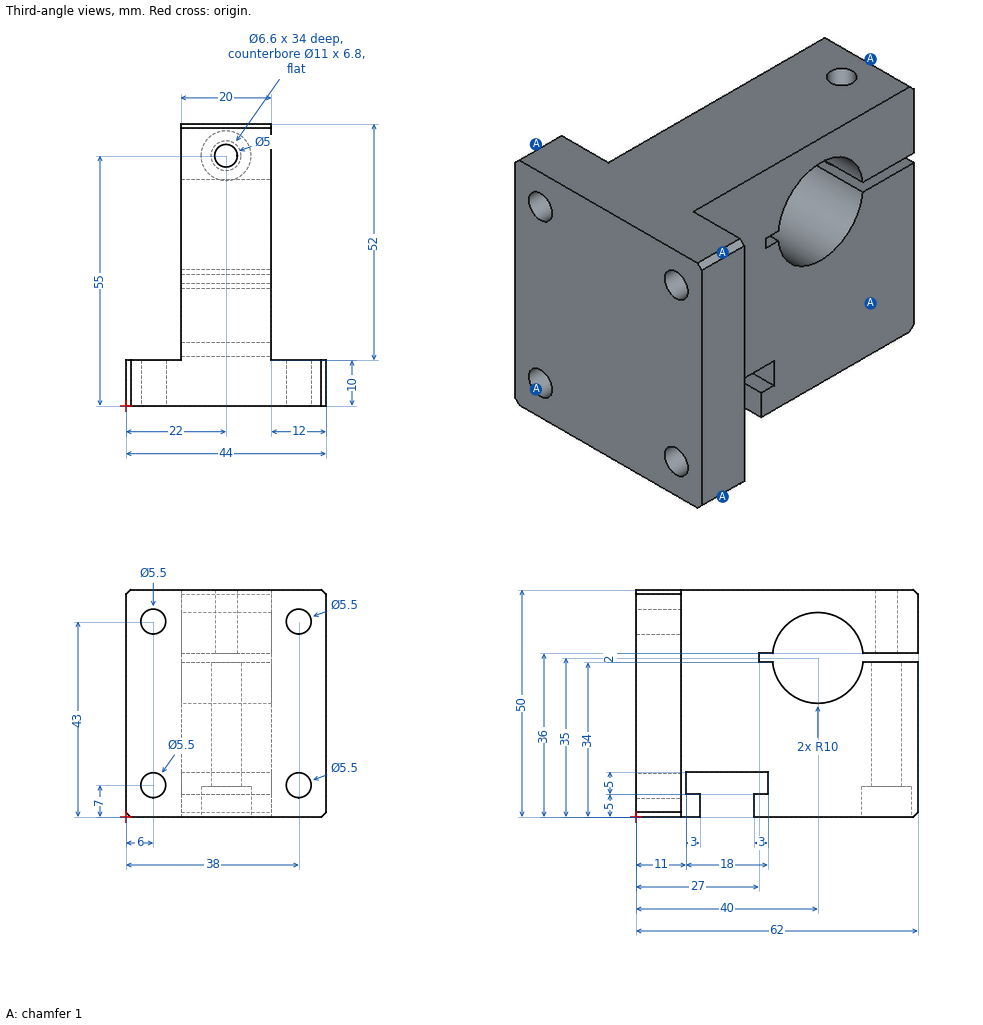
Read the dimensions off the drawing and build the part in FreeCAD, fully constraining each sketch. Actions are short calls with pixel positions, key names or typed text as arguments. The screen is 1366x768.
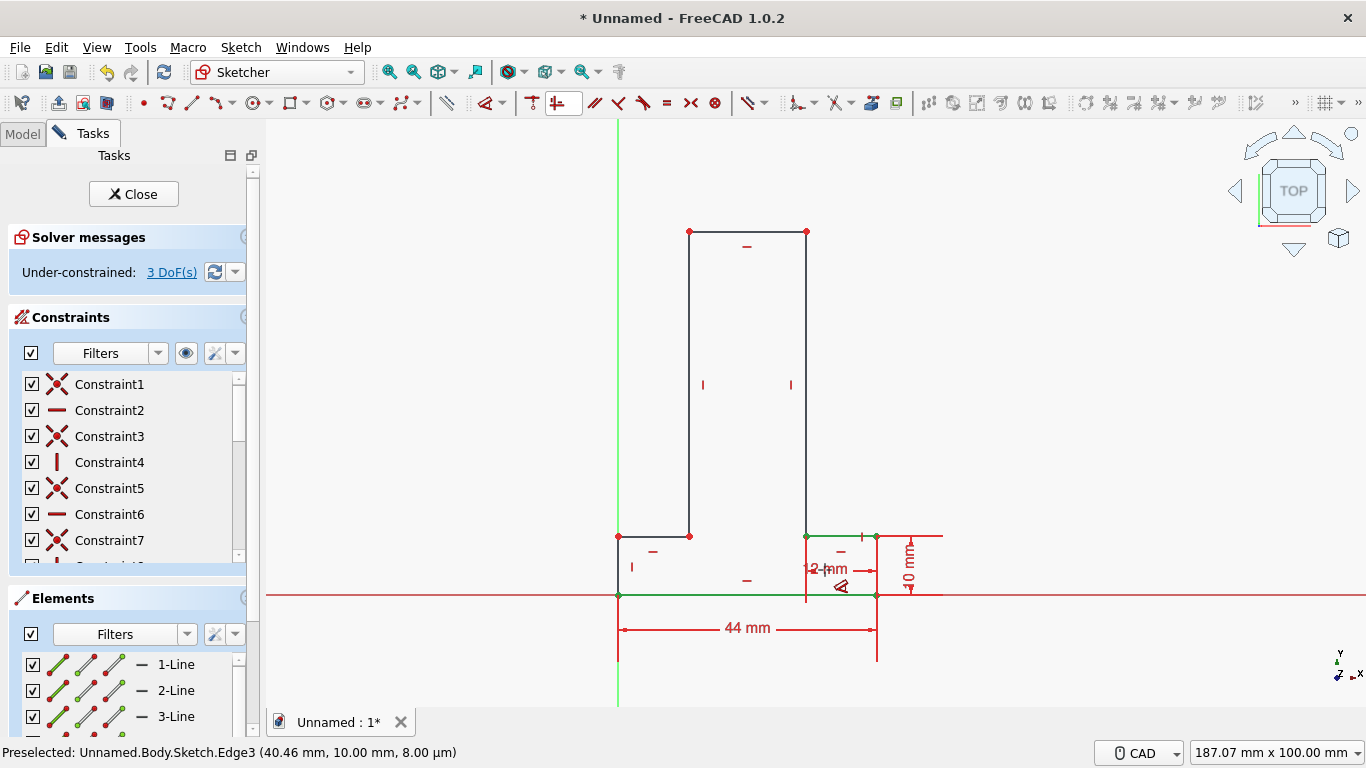
click(806, 445)
click(840, 384)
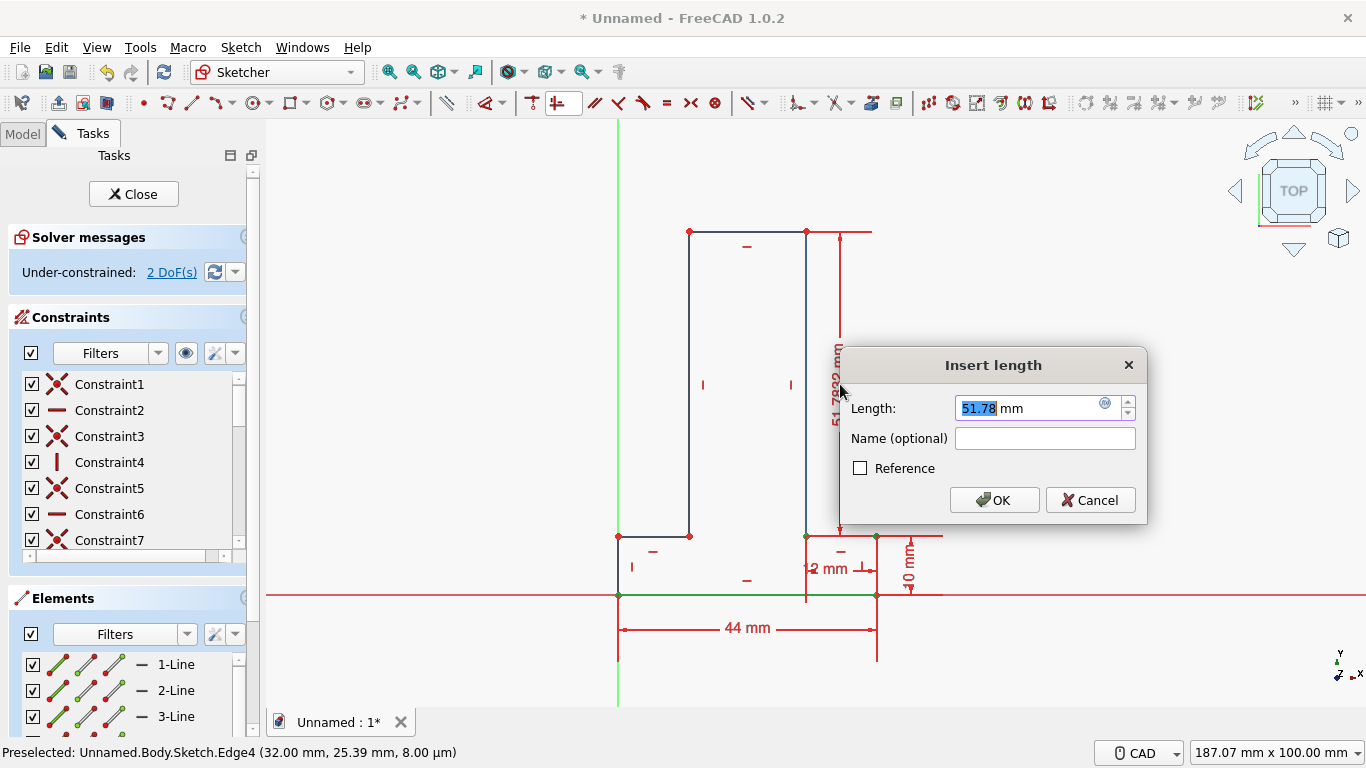
text(52)
key(Return)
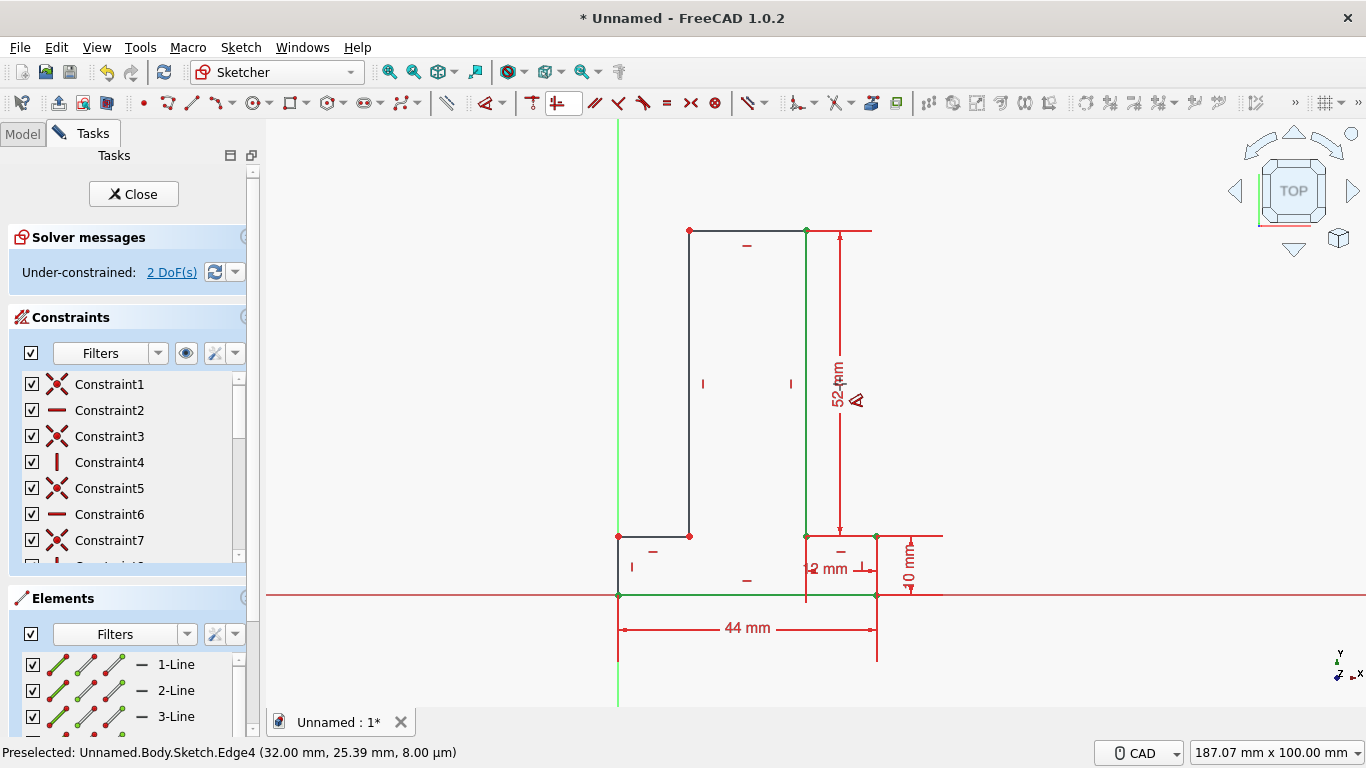
click(771, 231)
click(748, 197)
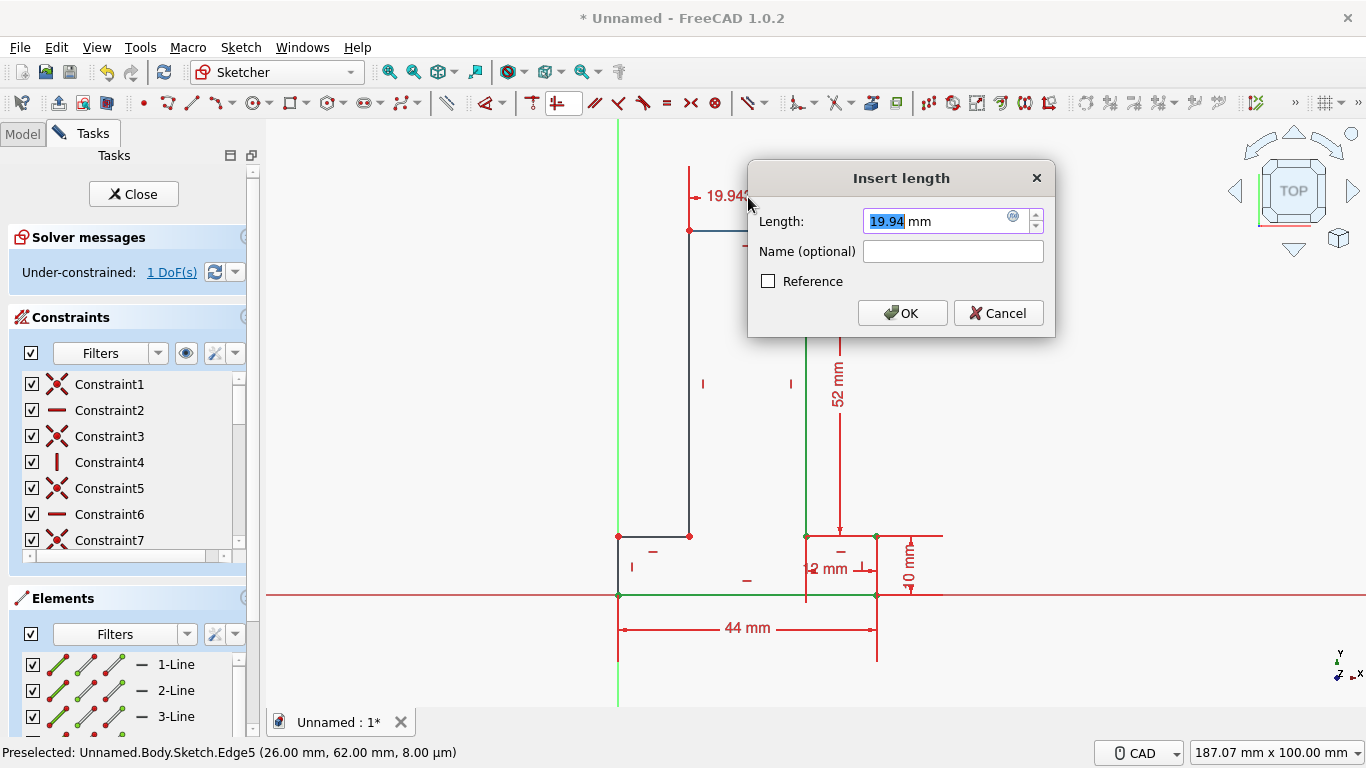
text(20)
key(Return)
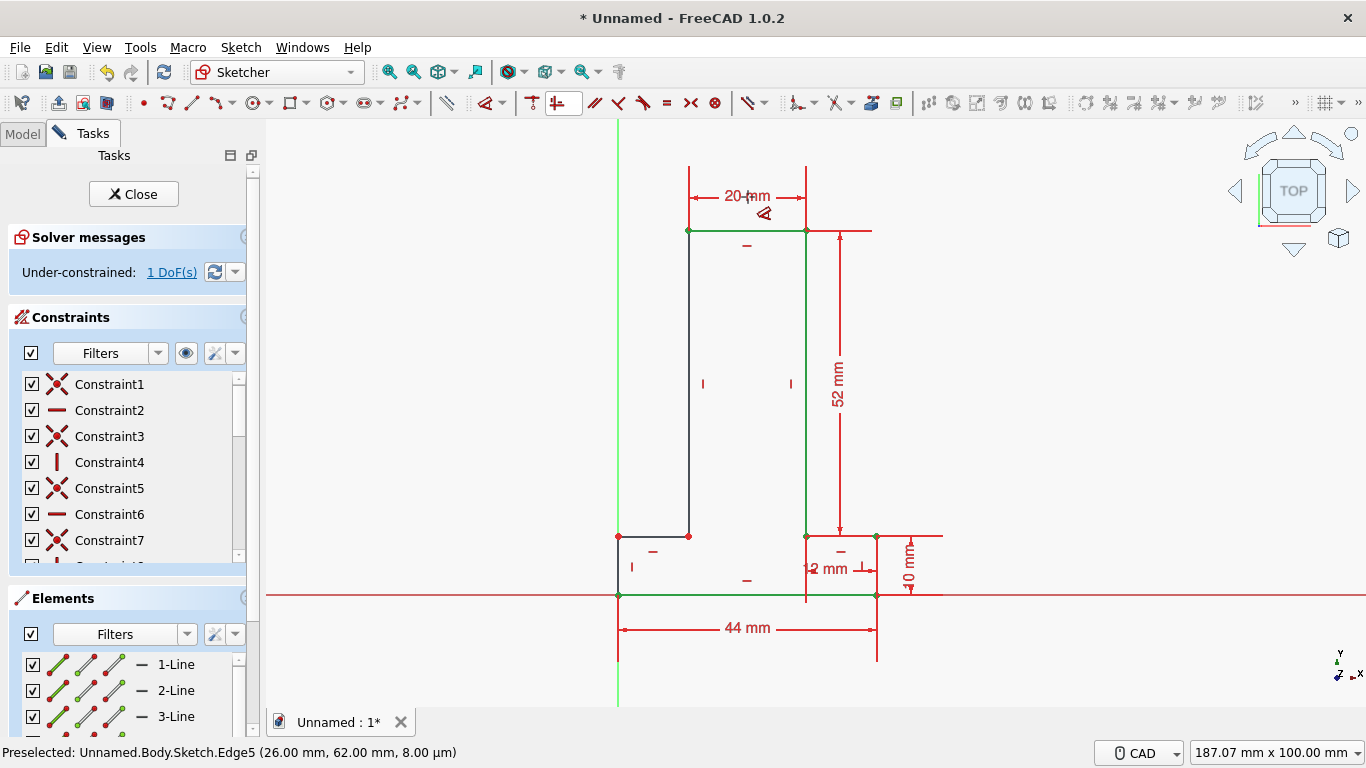
click(689, 323)
click(655, 384)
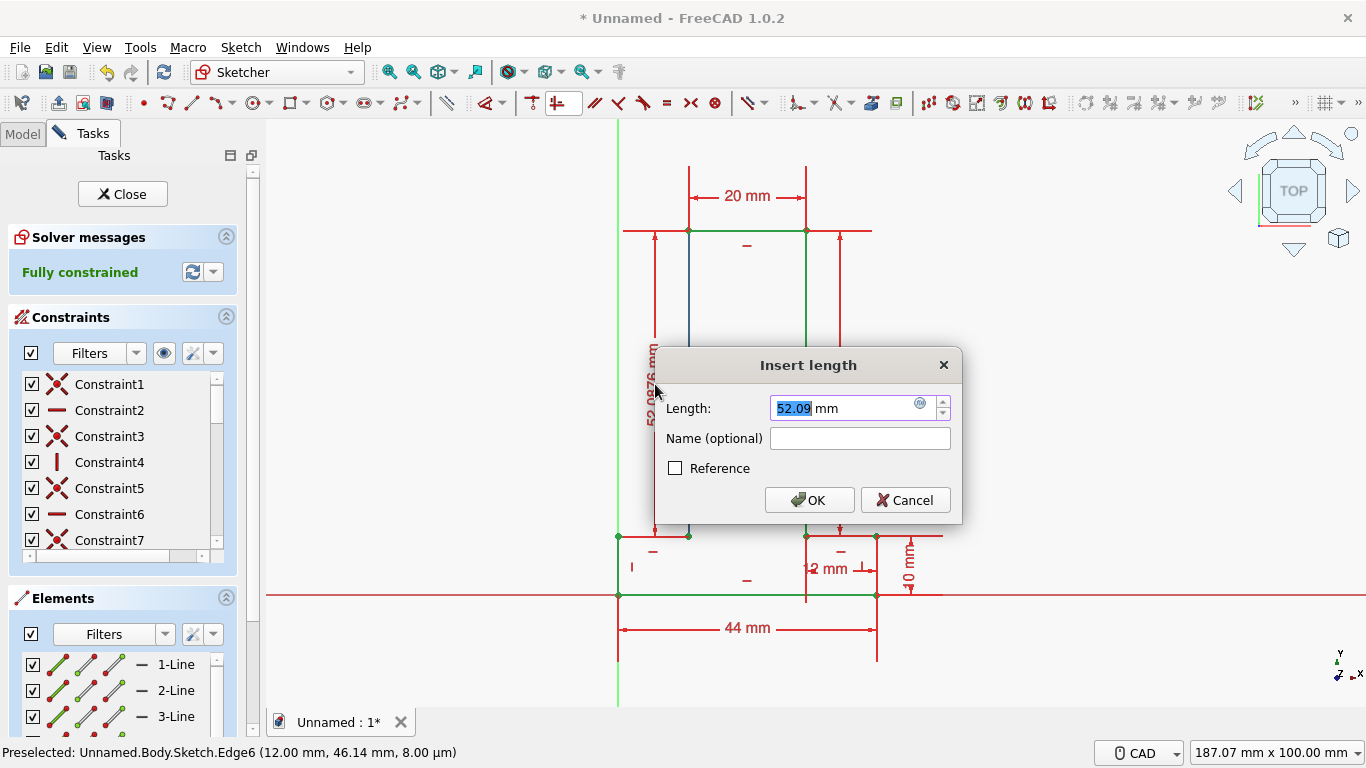
text(52)
key(Return)
key(Escape)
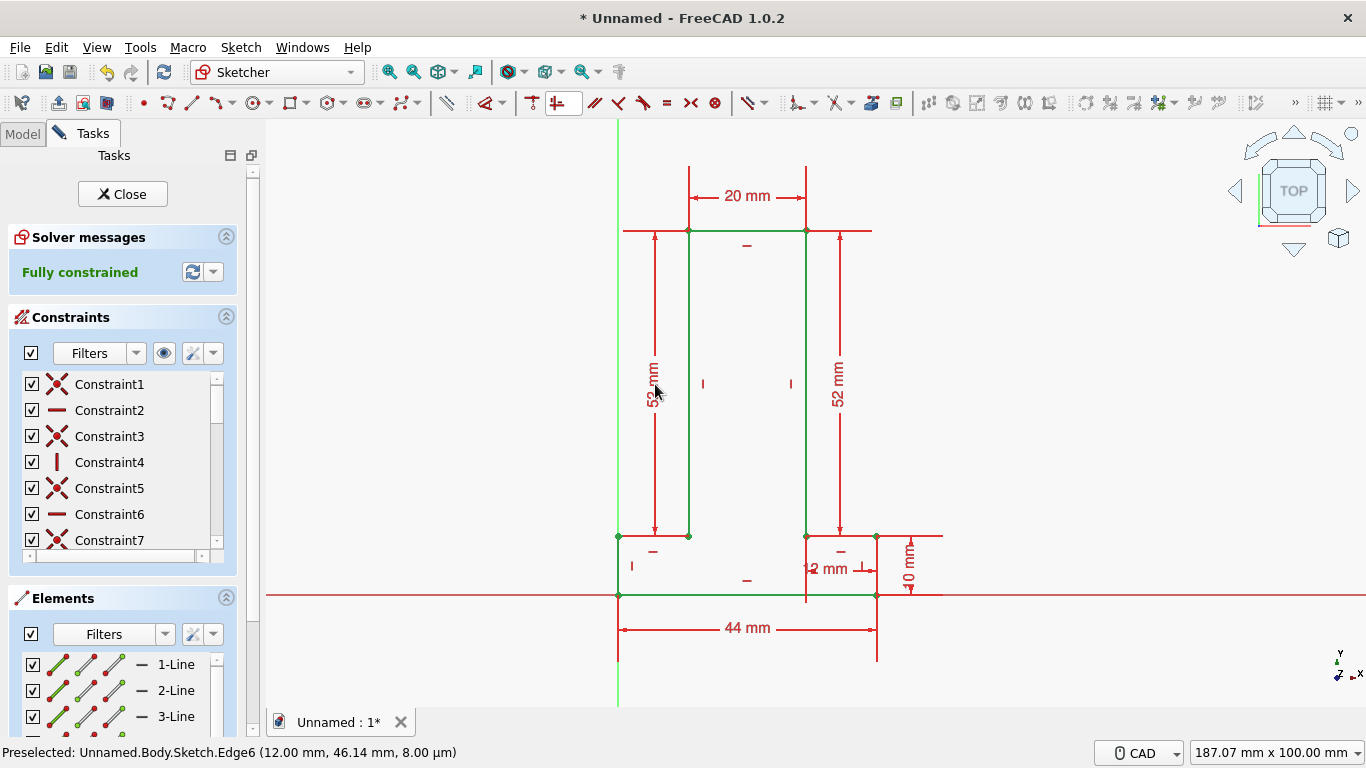
click(123, 194)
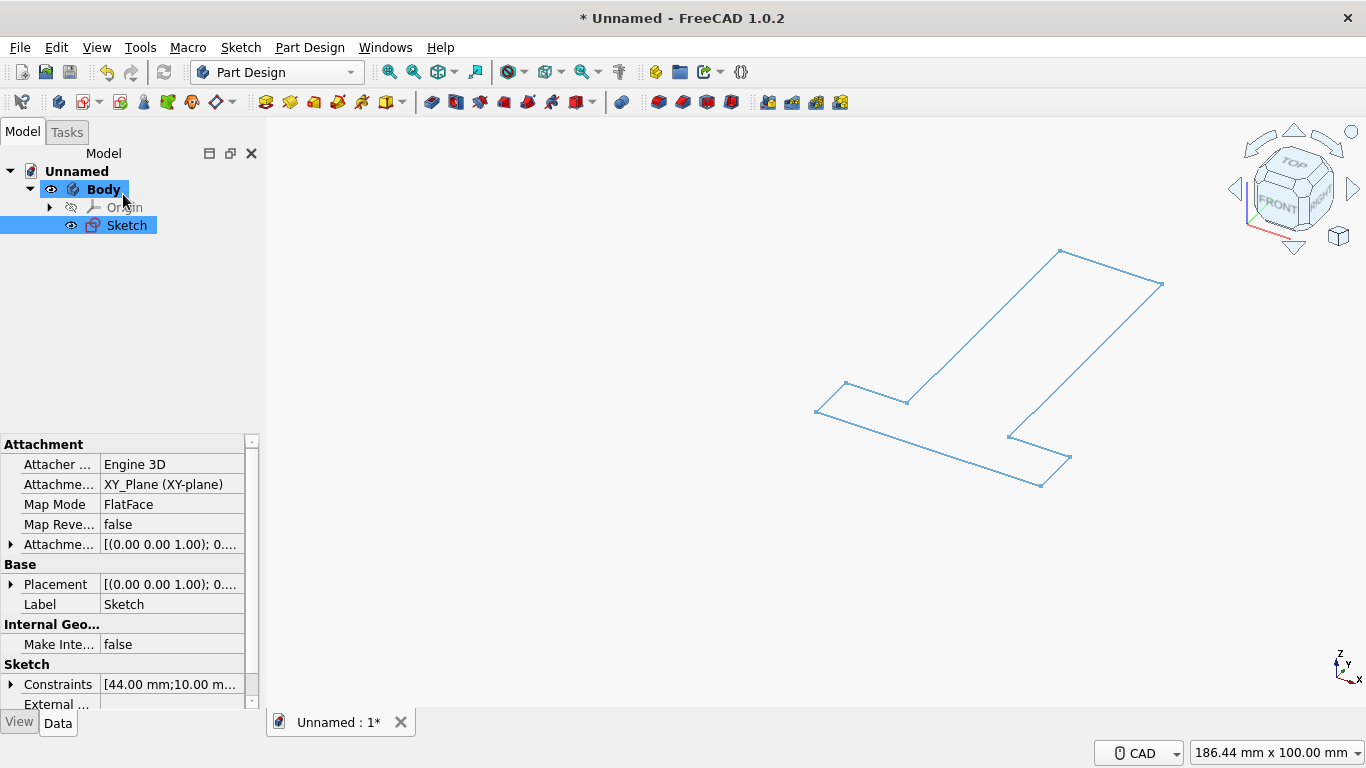
click(266, 102)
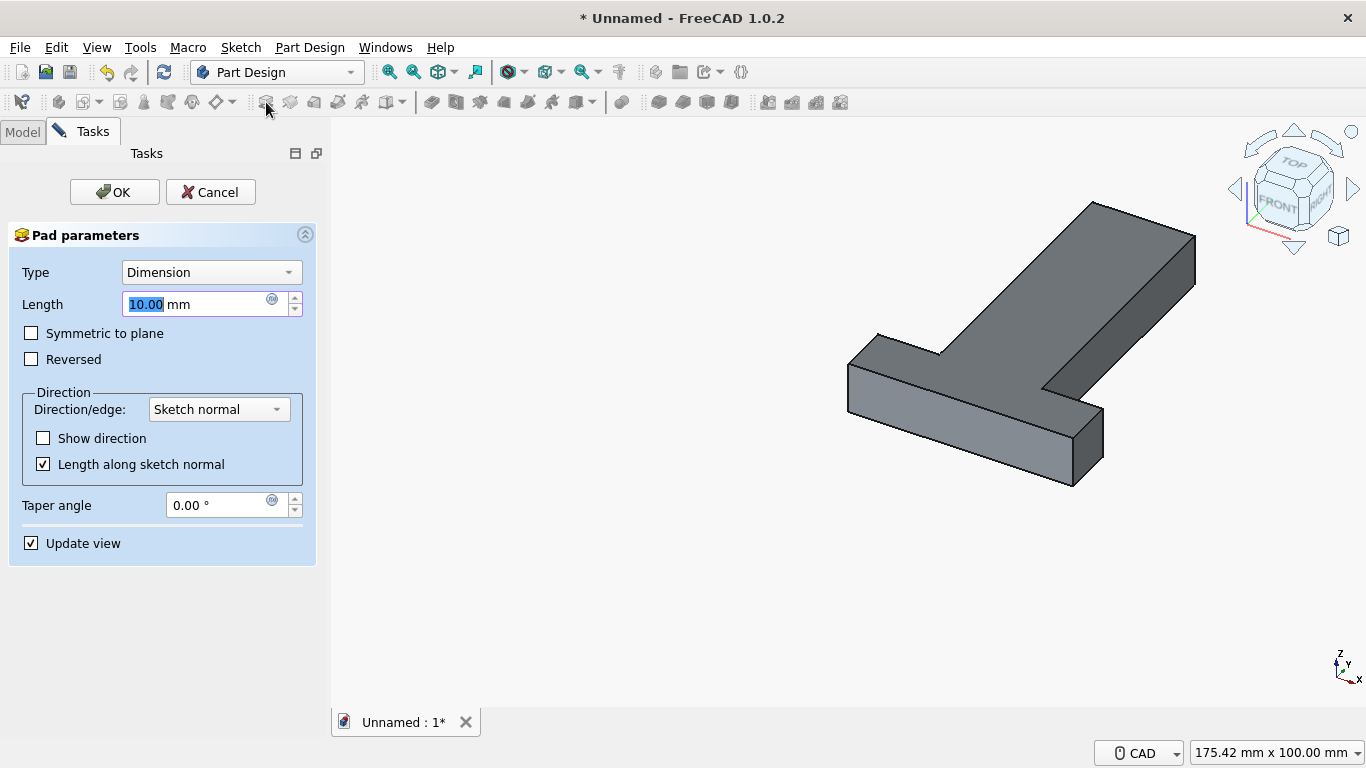
text(50)
key(Tab)